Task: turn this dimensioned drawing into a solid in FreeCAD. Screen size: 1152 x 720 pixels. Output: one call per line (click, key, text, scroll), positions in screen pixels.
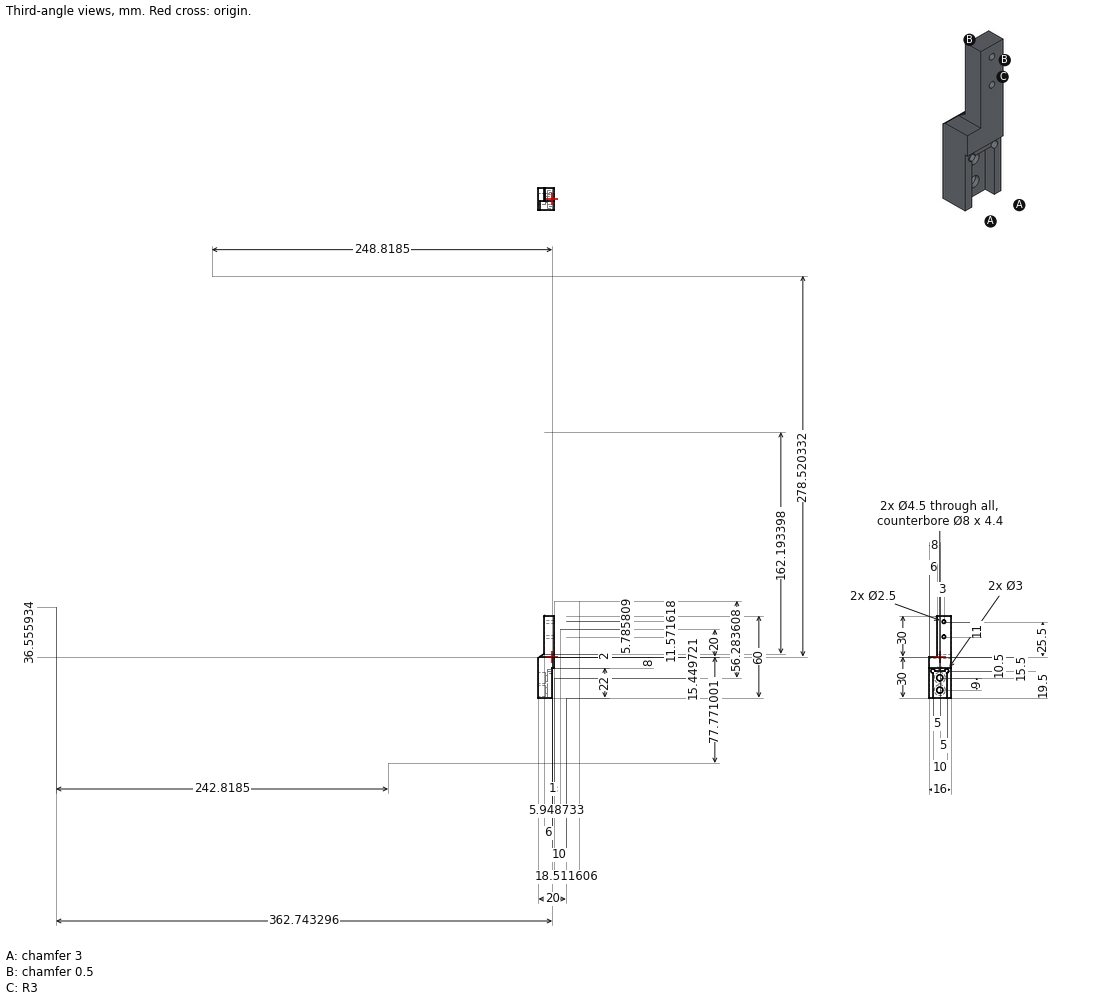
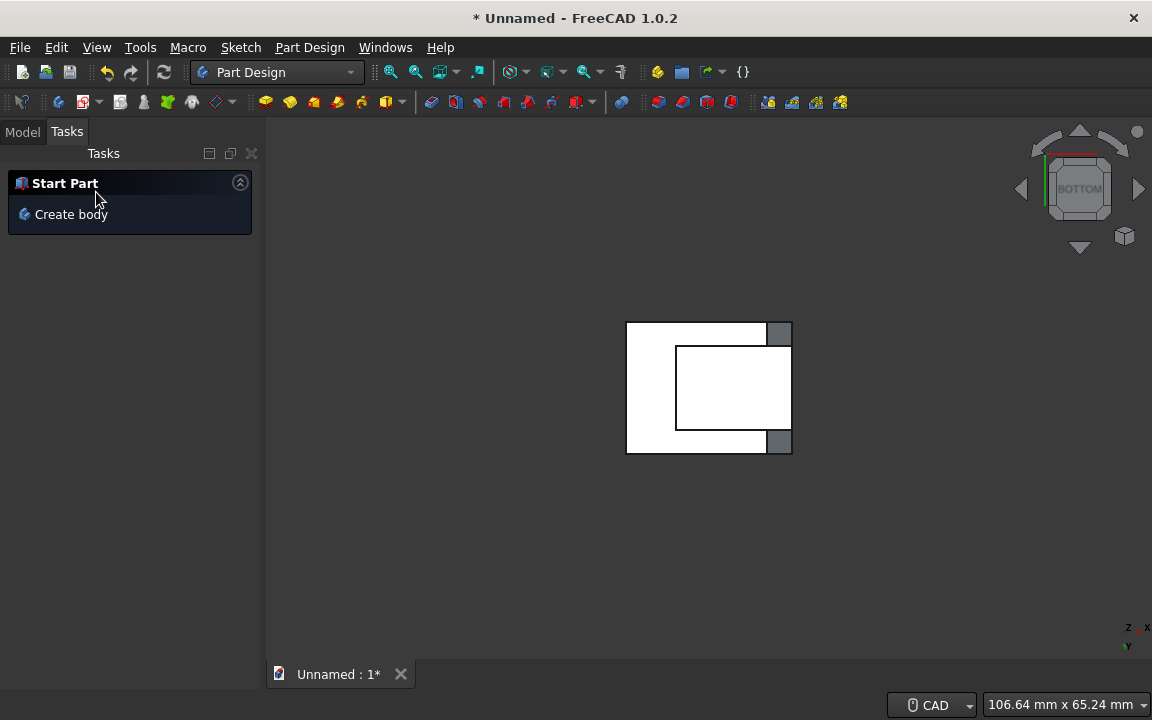
key(v)
key(f)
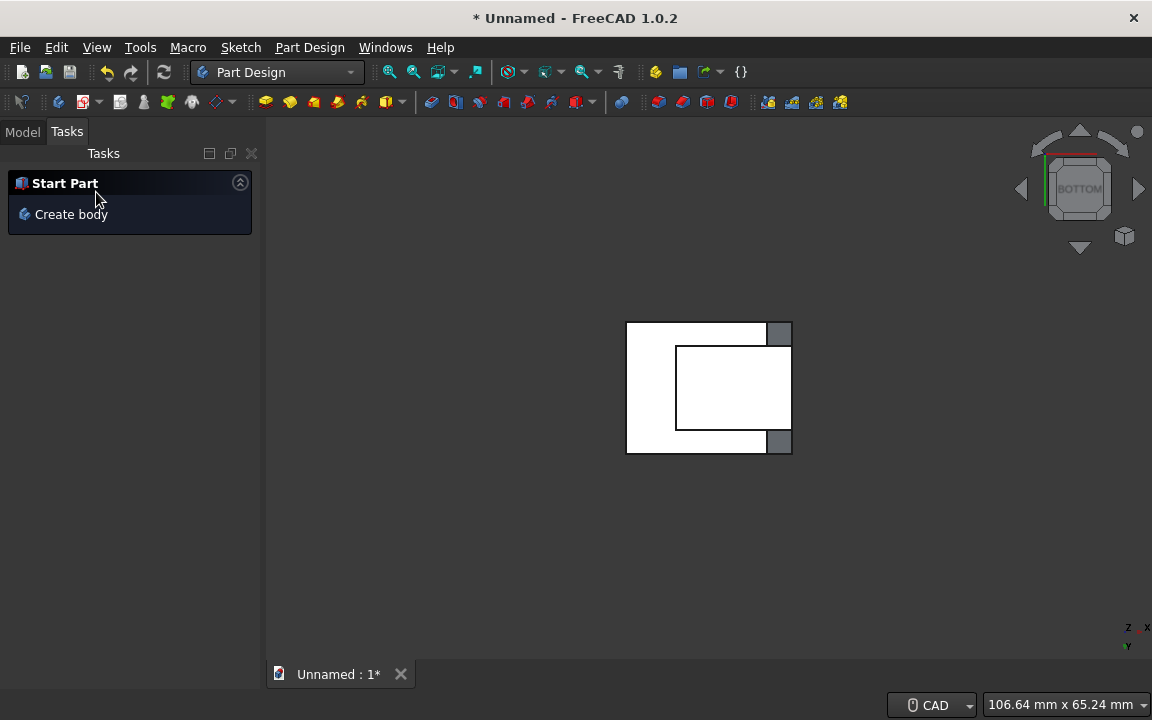
key(0)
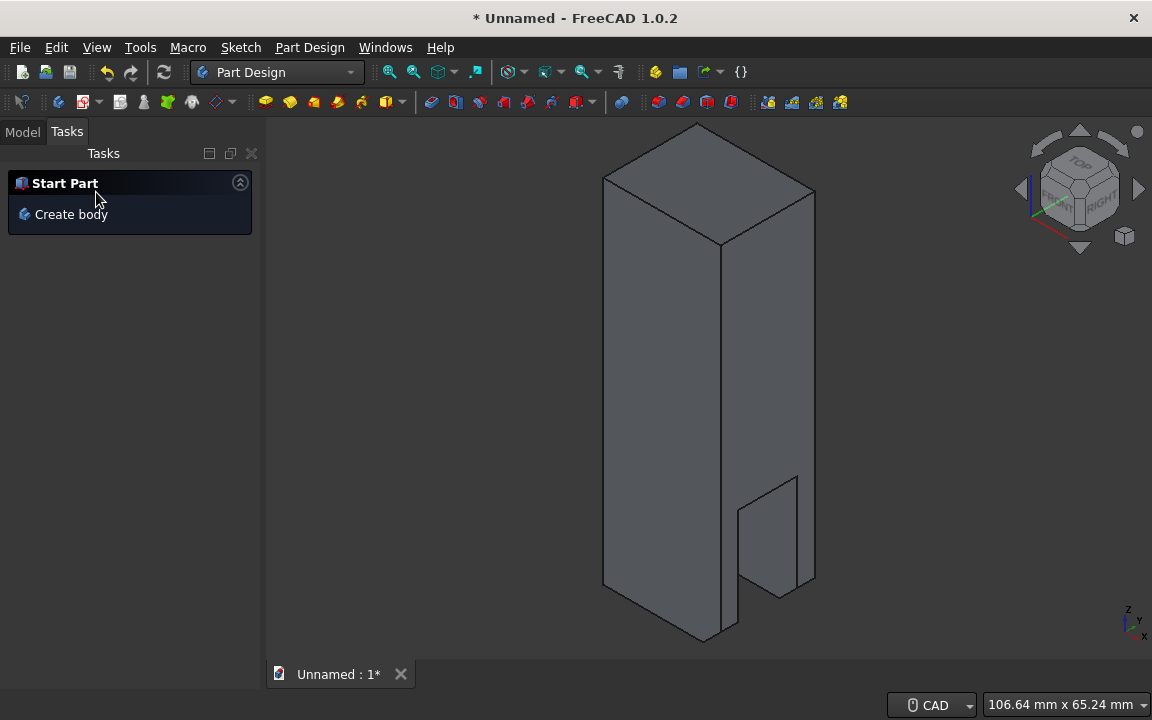
click(662, 298)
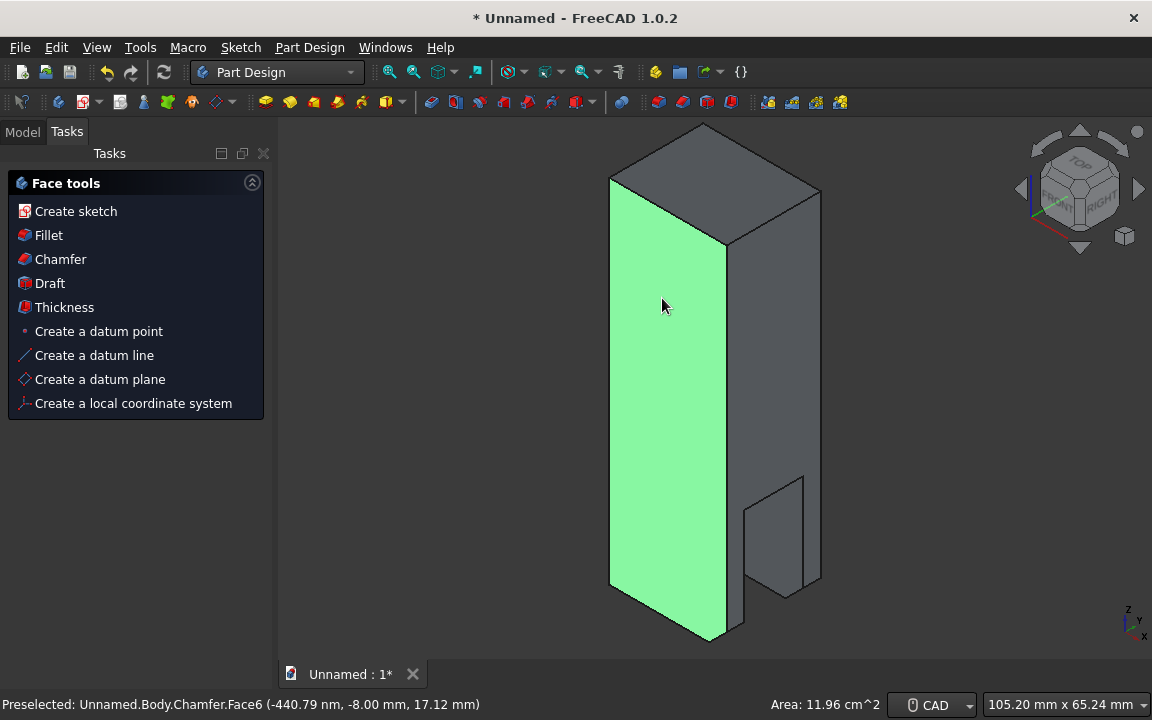
click(84, 102)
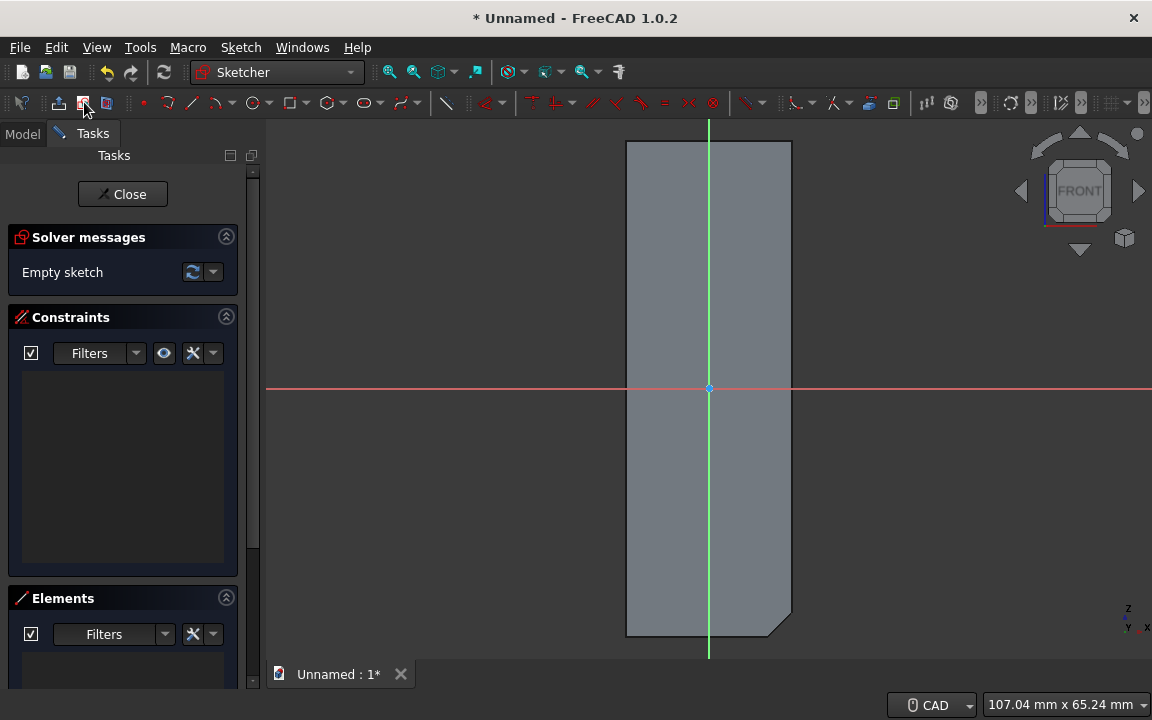
scroll(819, 493, down, 11)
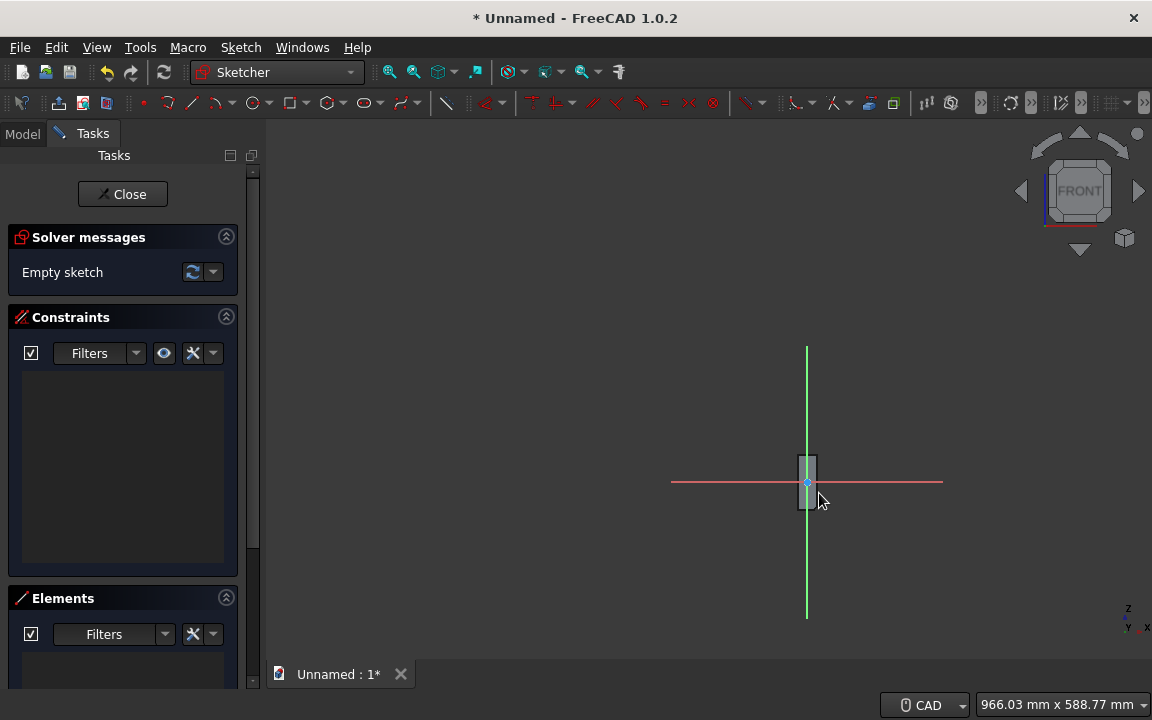
key(g)
key(m)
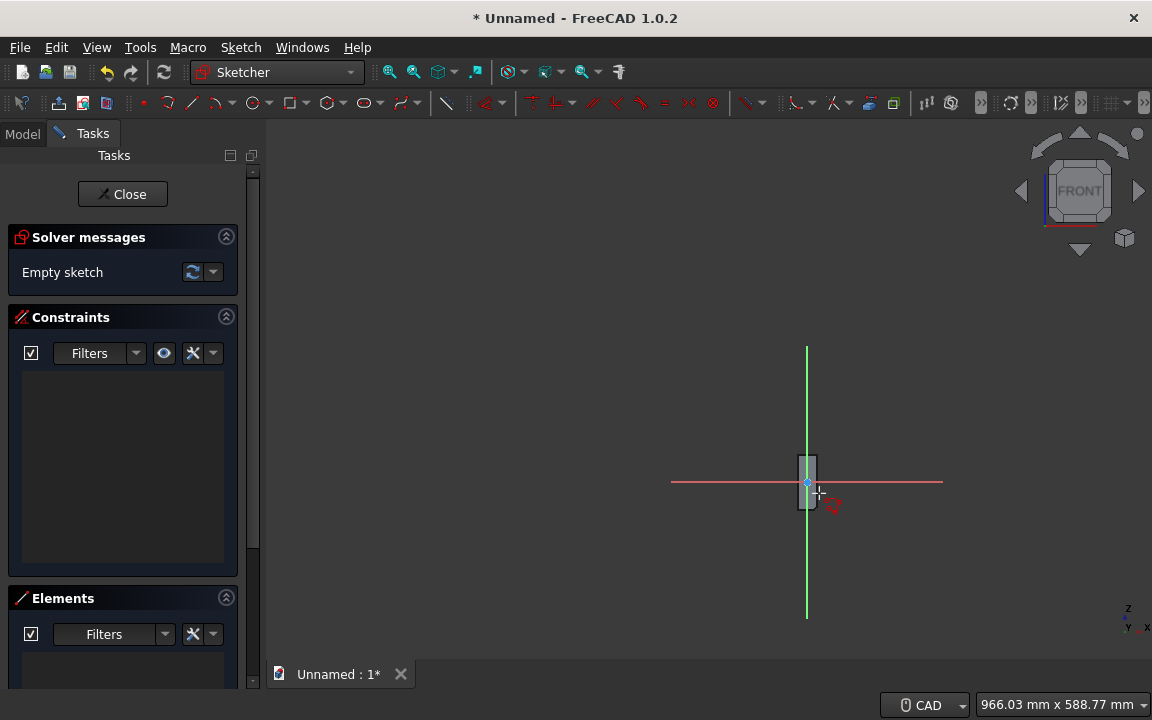
scroll(802, 480, up, 11)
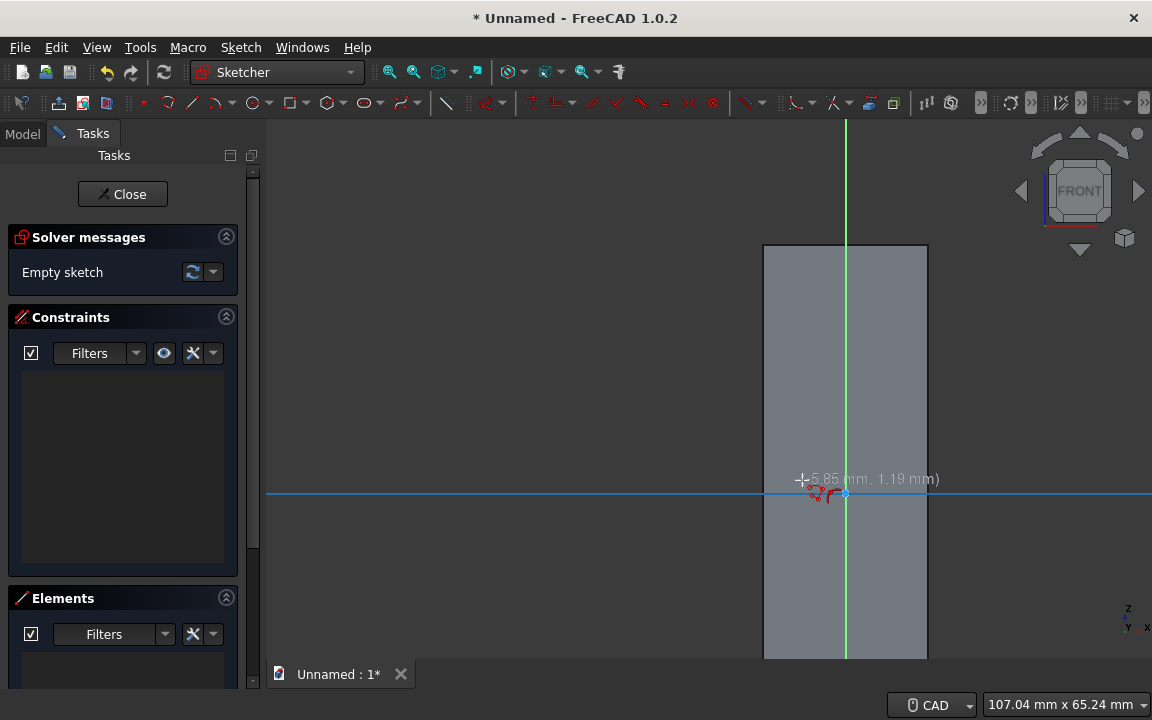
click(796, 477)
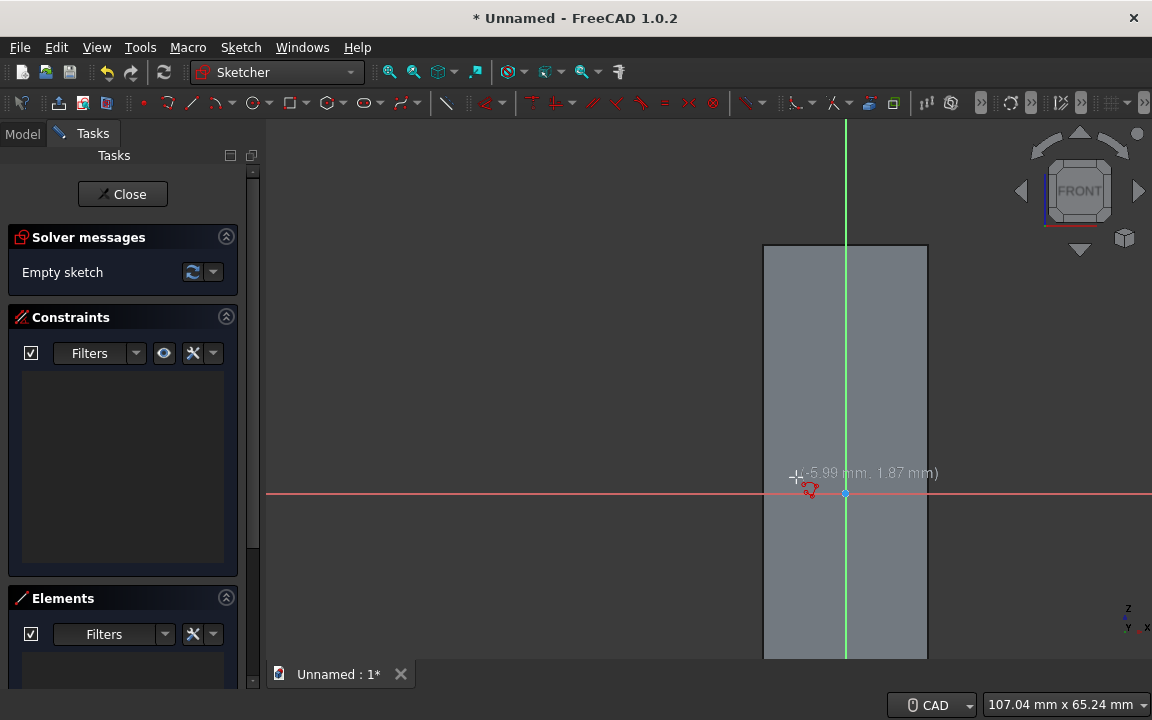
scroll(802, 480, down, 11)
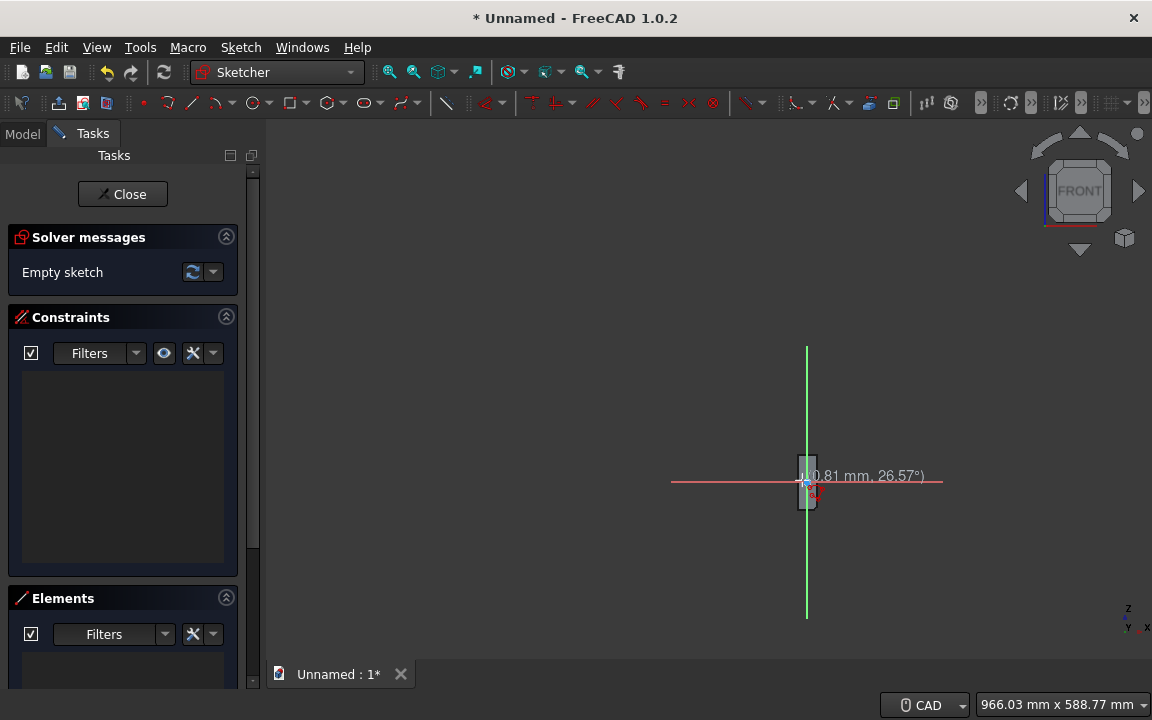
scroll(802, 332, up, 6)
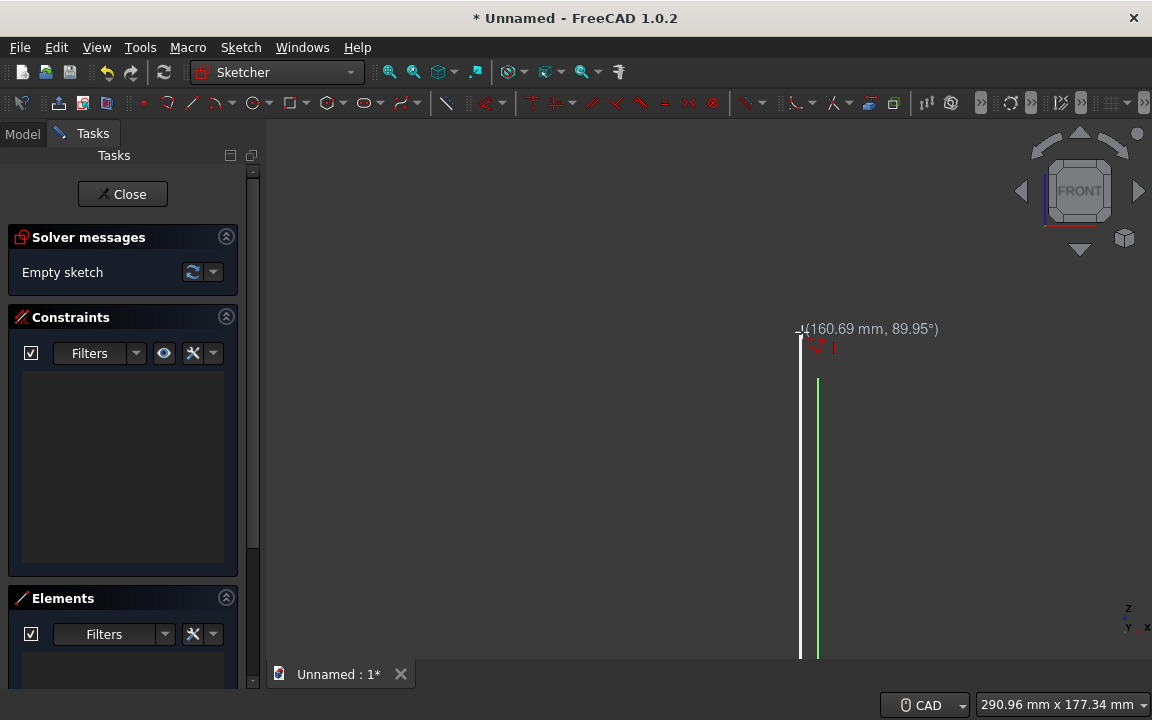
click(800, 329)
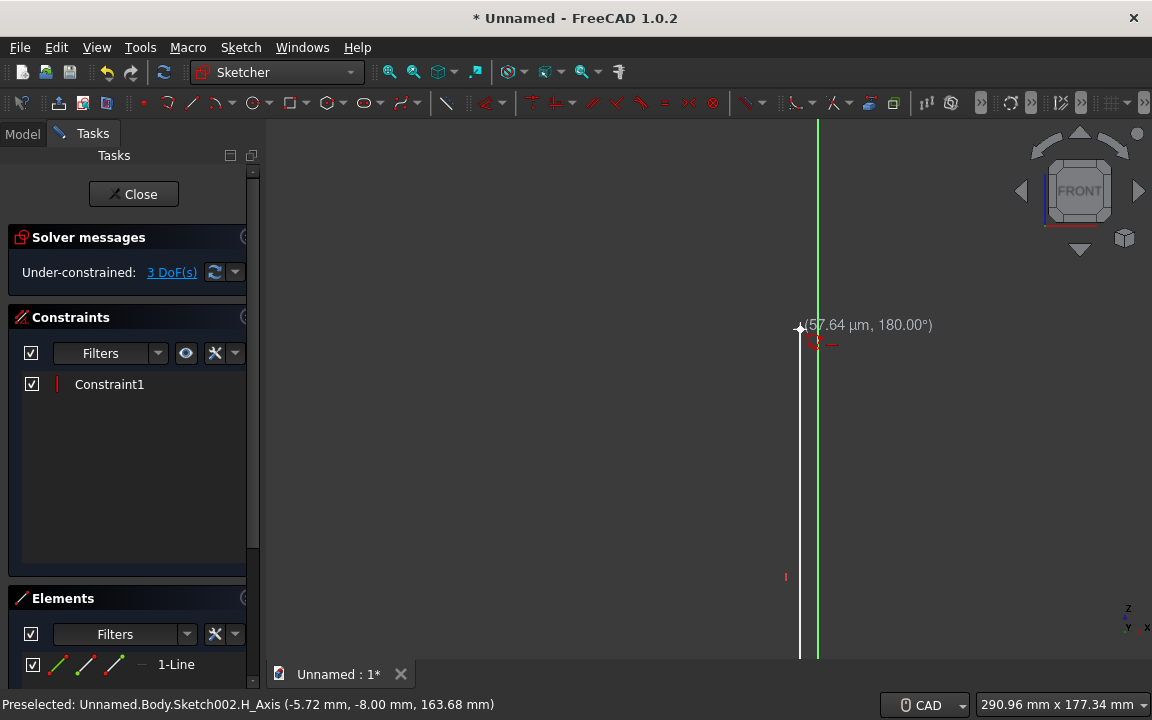
scroll(802, 331, down, 6)